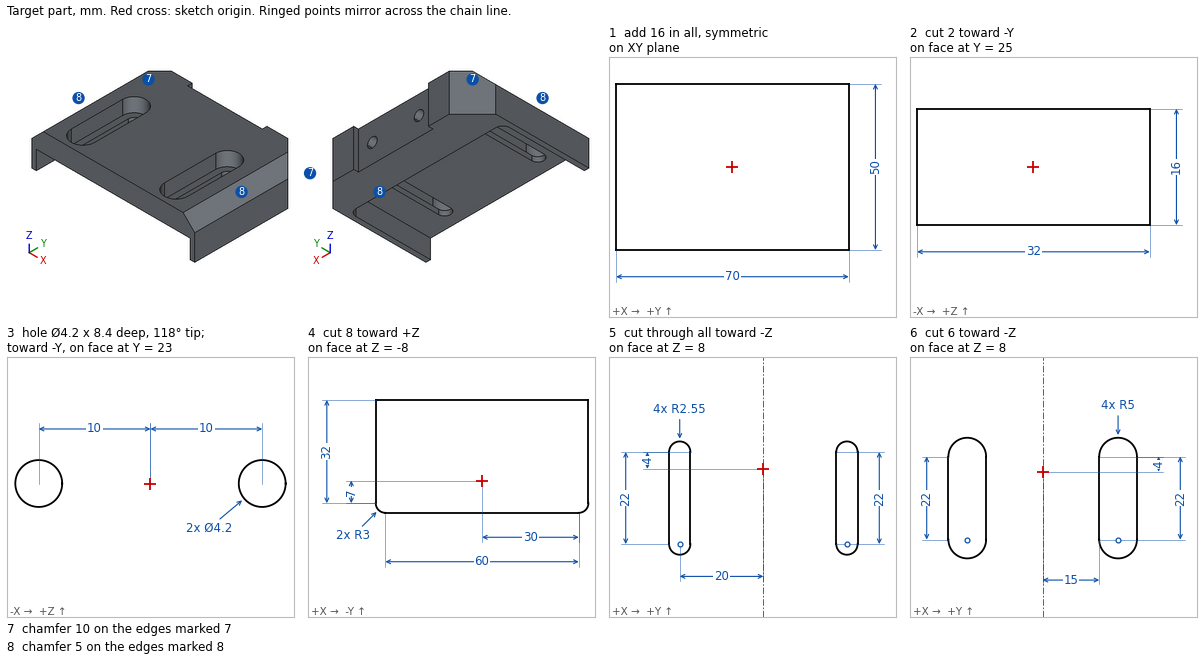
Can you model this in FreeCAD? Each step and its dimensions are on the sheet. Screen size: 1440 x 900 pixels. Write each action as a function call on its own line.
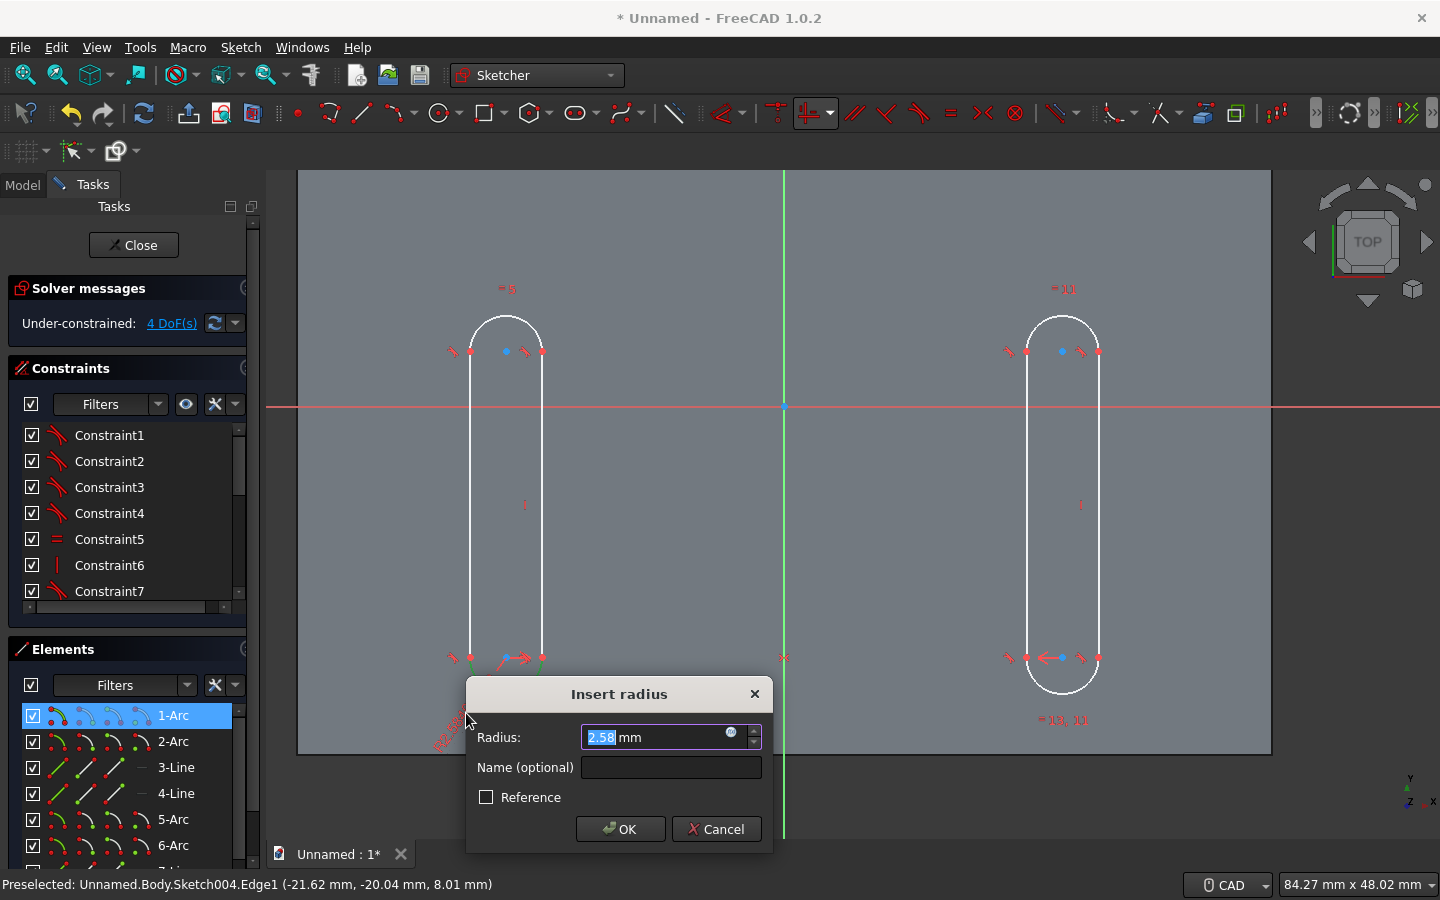
text(2.55)
key(Return)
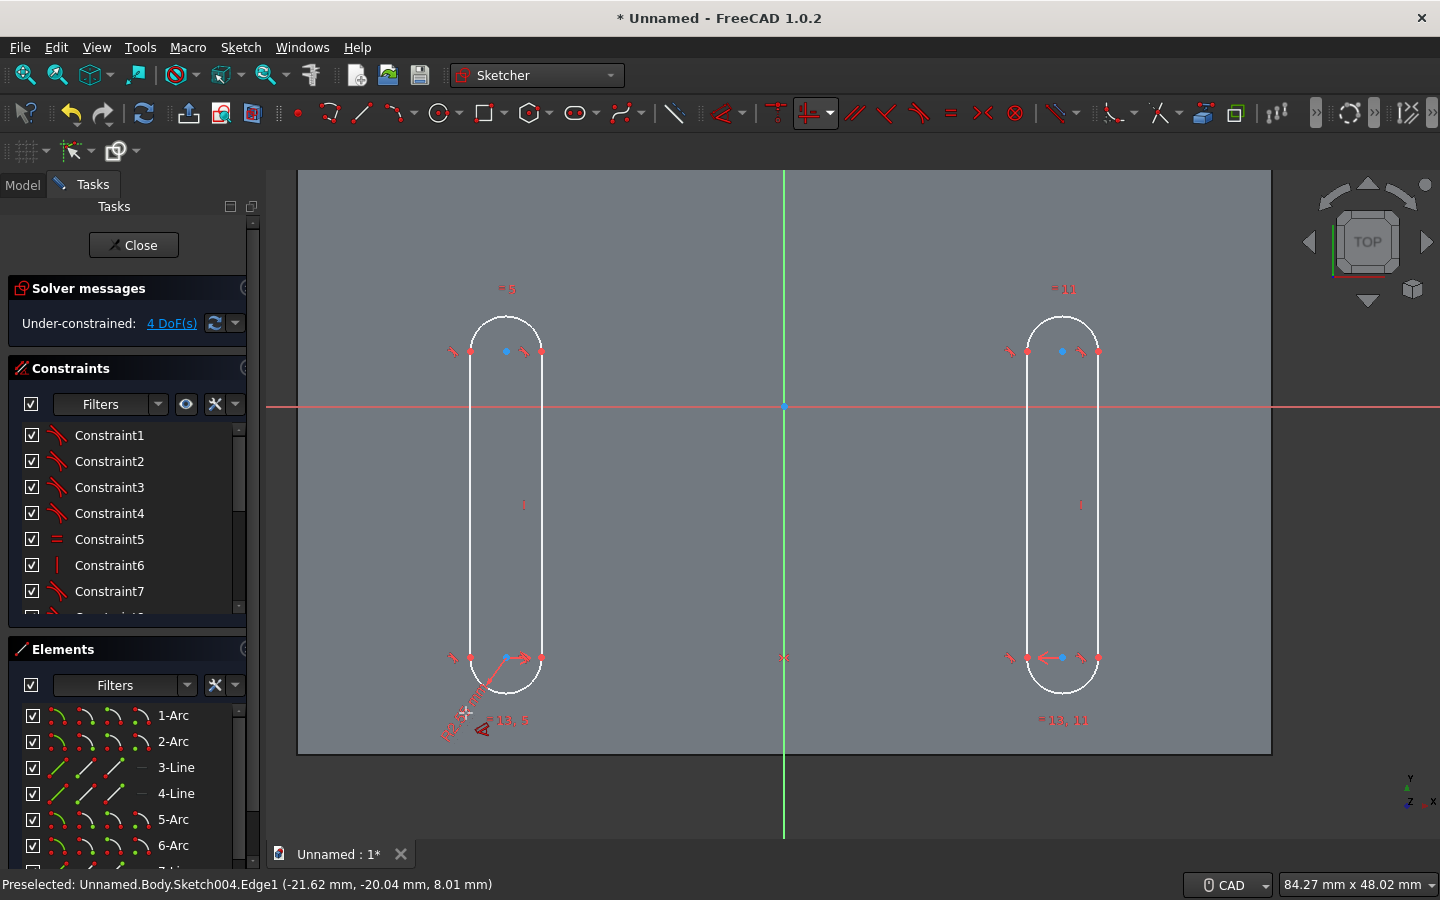
click(470, 566)
click(436, 505)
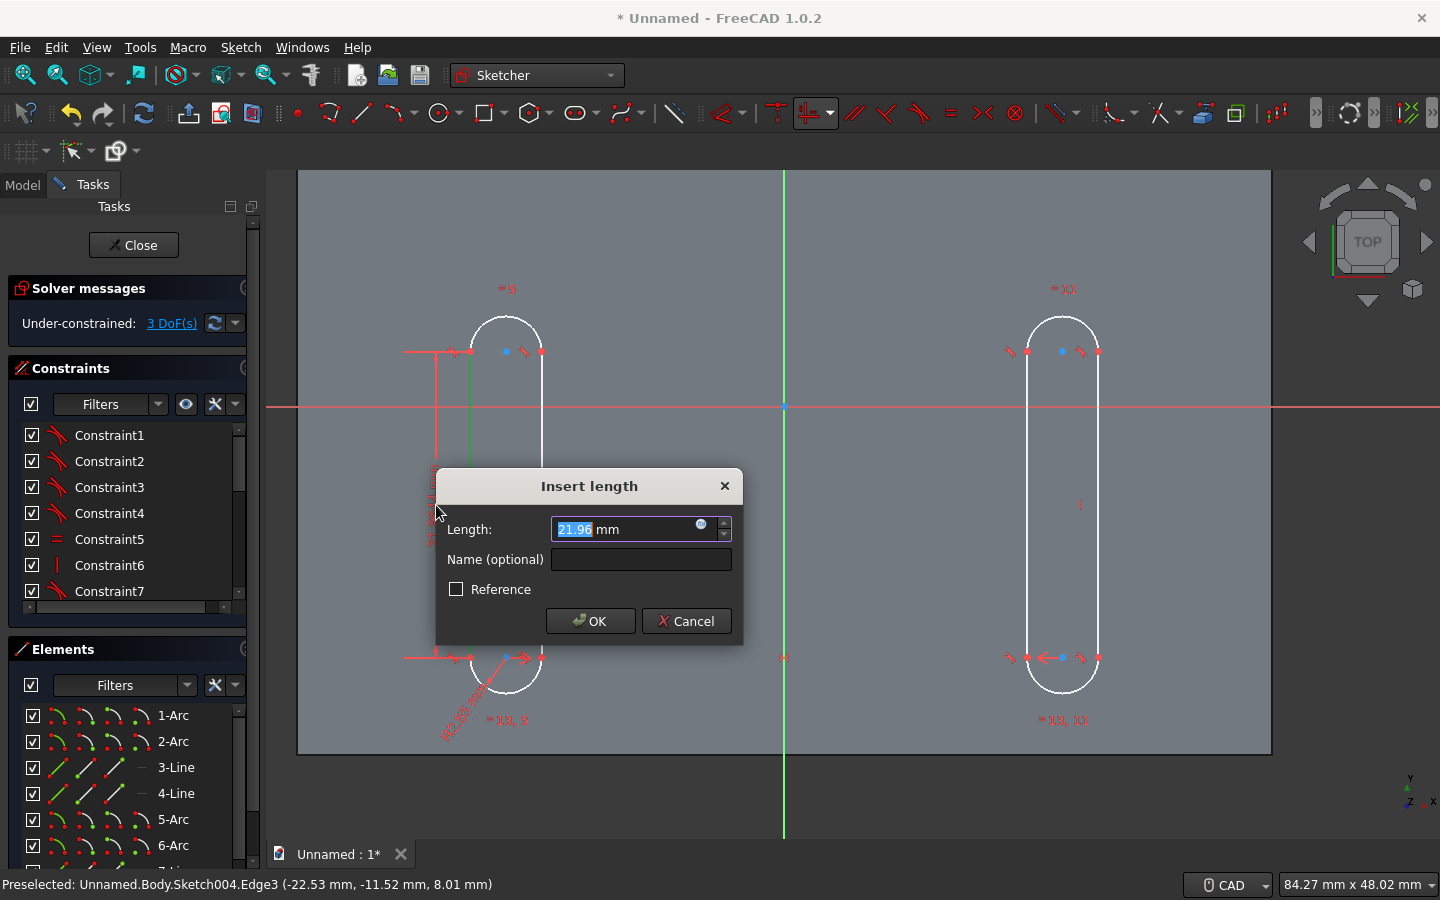
text(22)
key(Return)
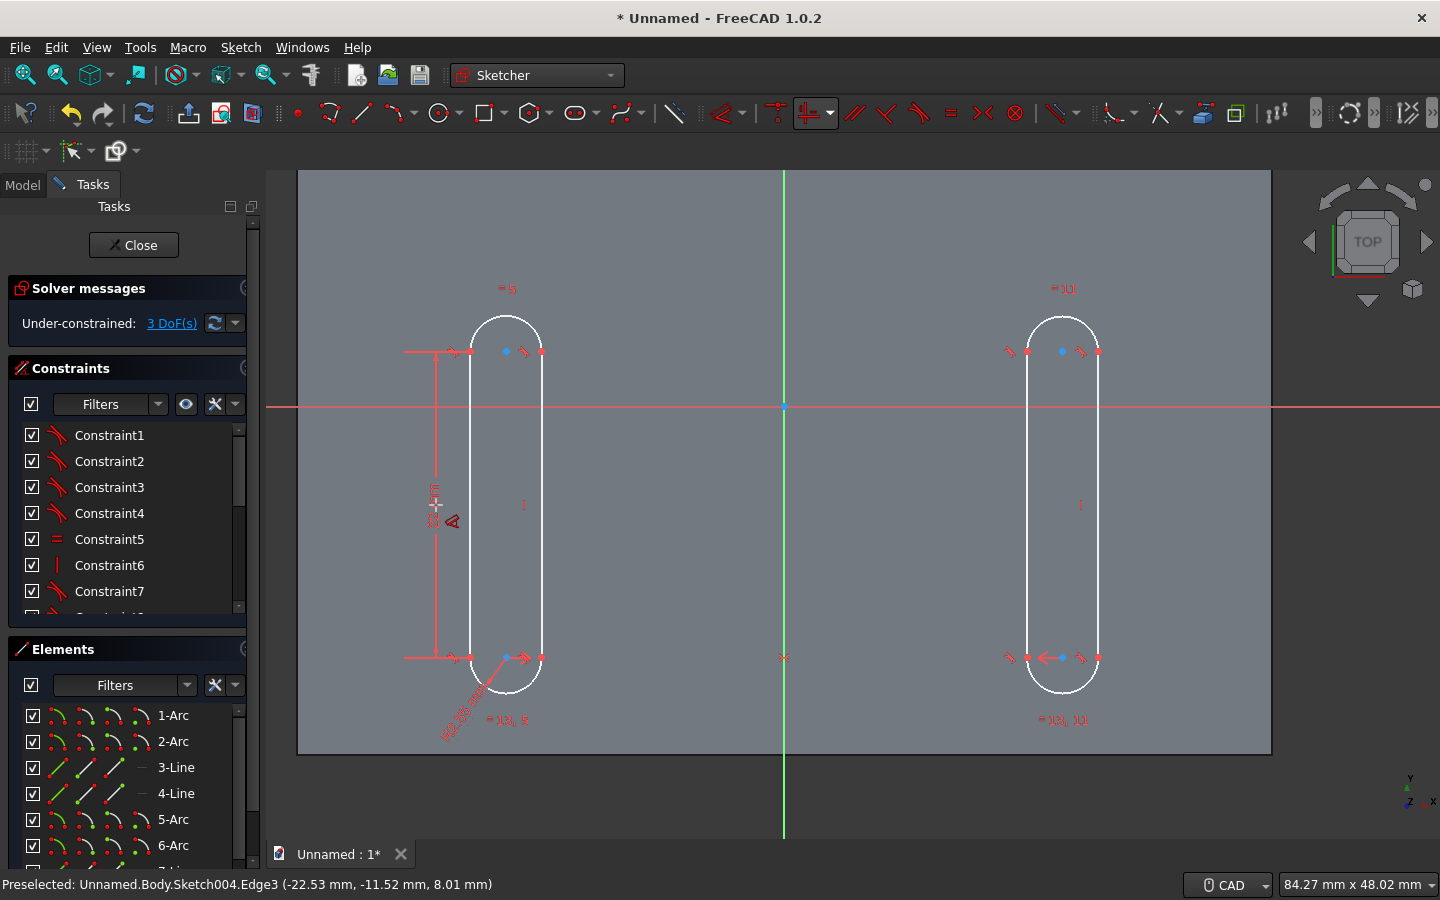
click(1027, 566)
click(1061, 505)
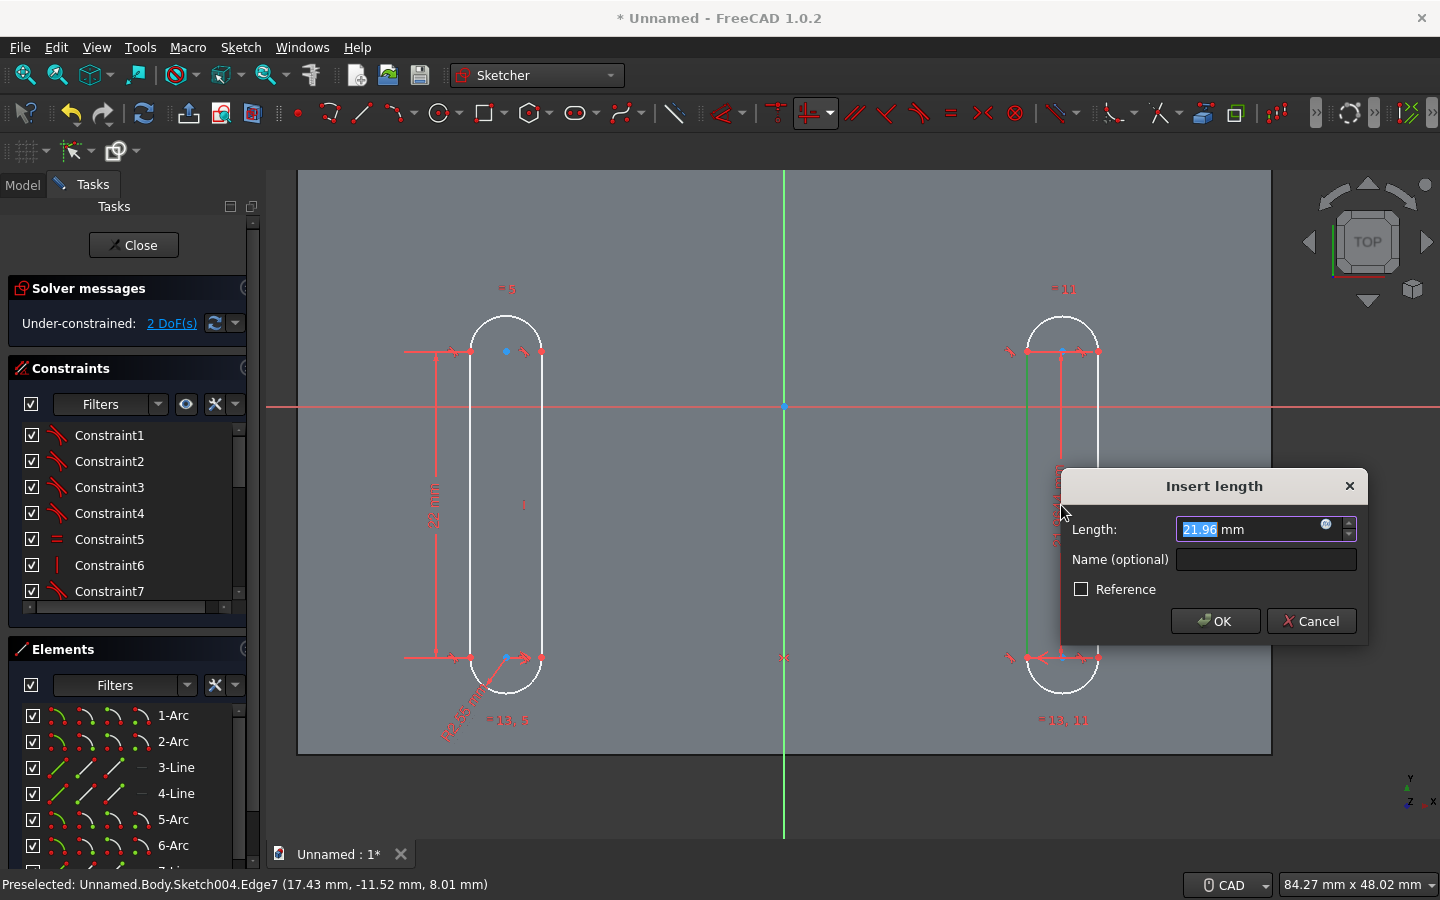
text(22)
key(Return)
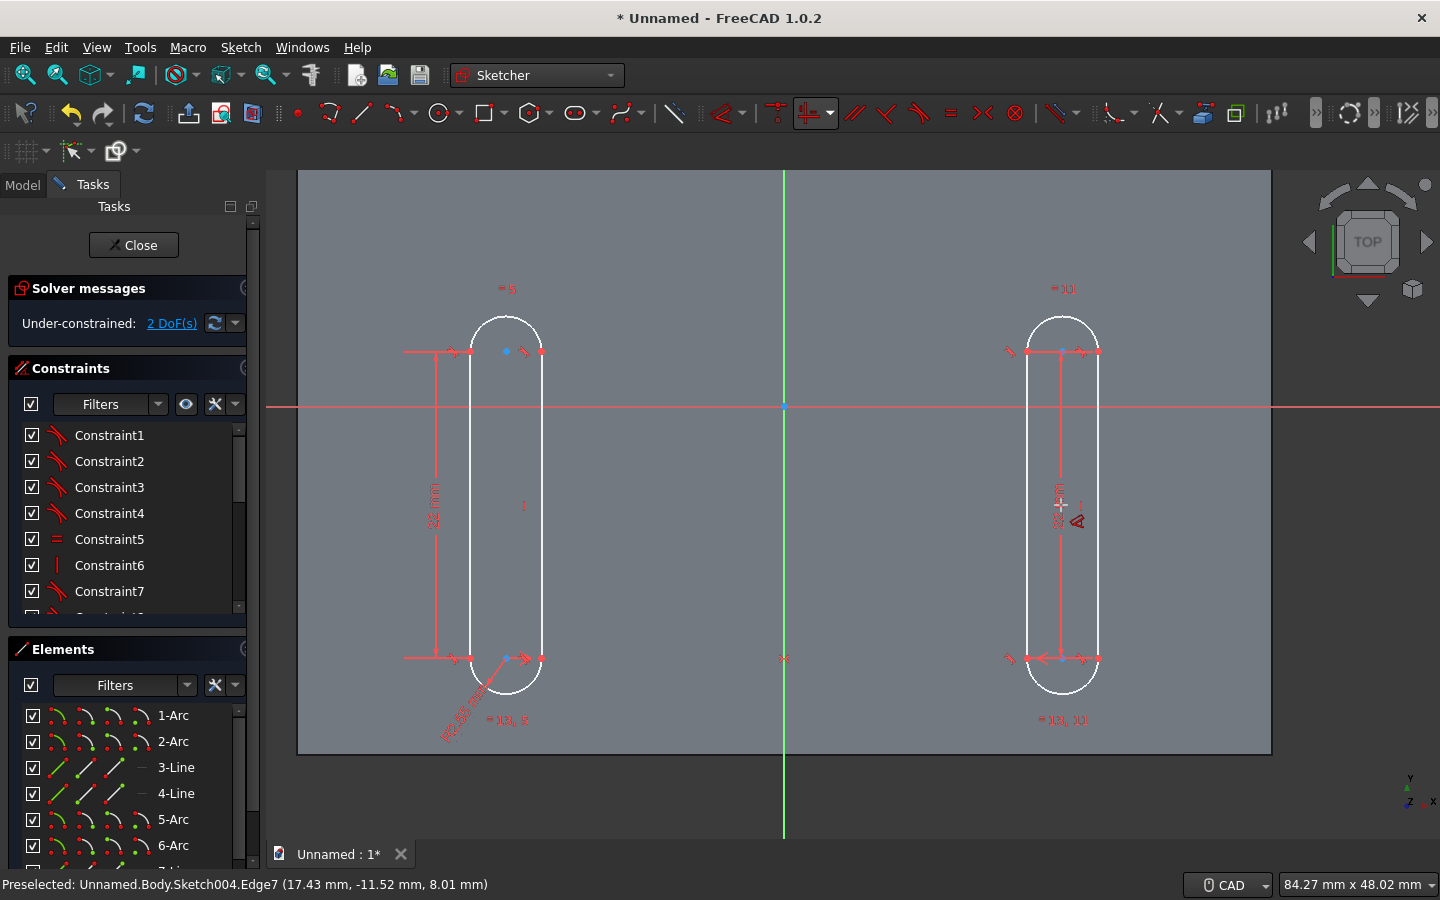
click(542, 352)
click(508, 379)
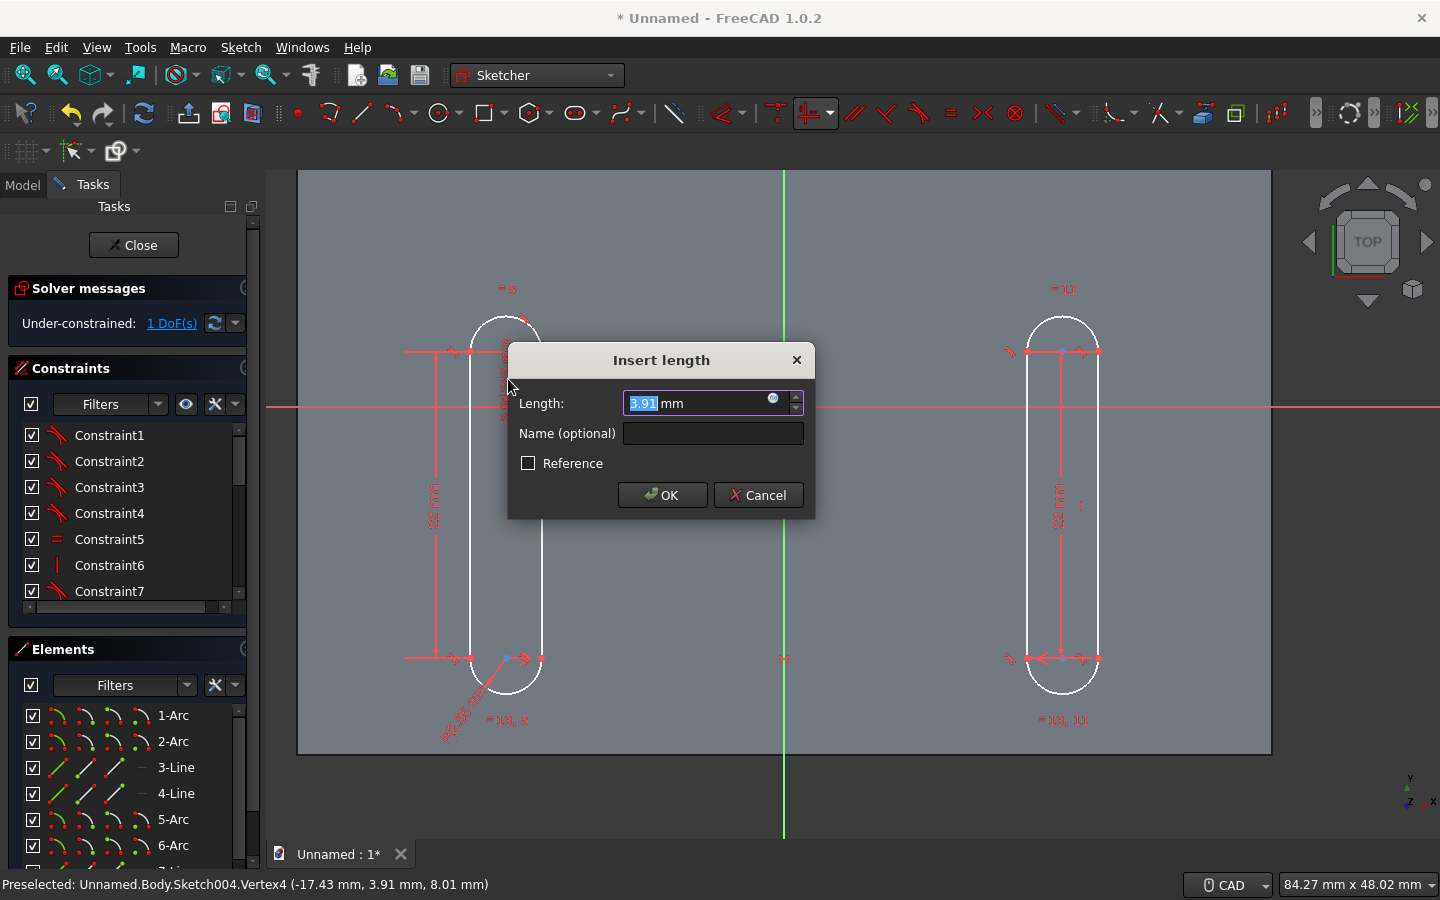
text(4)
key(Return)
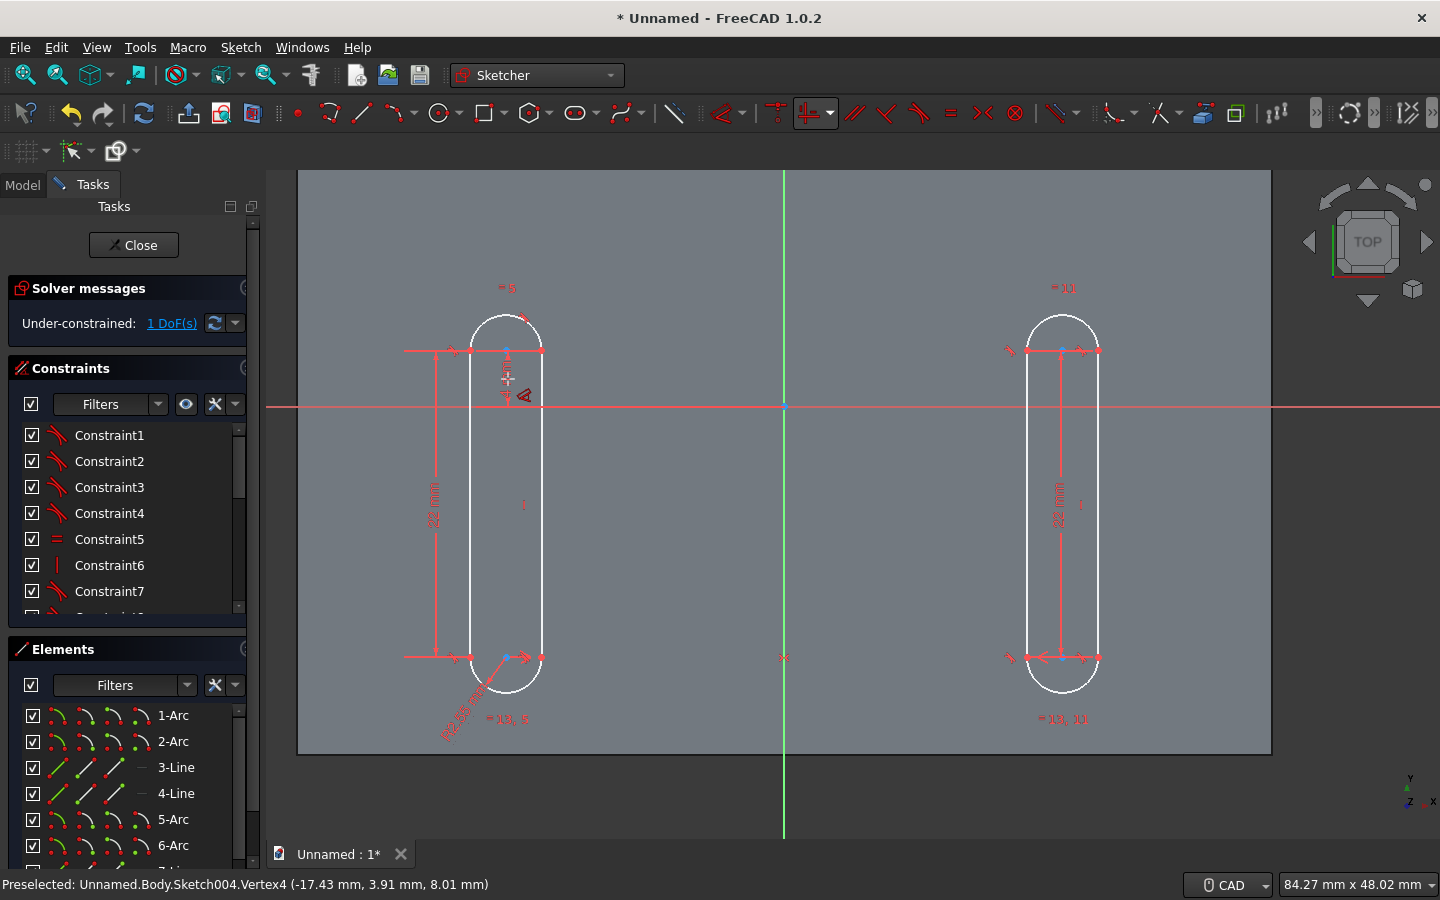
click(506, 657)
click(645, 691)